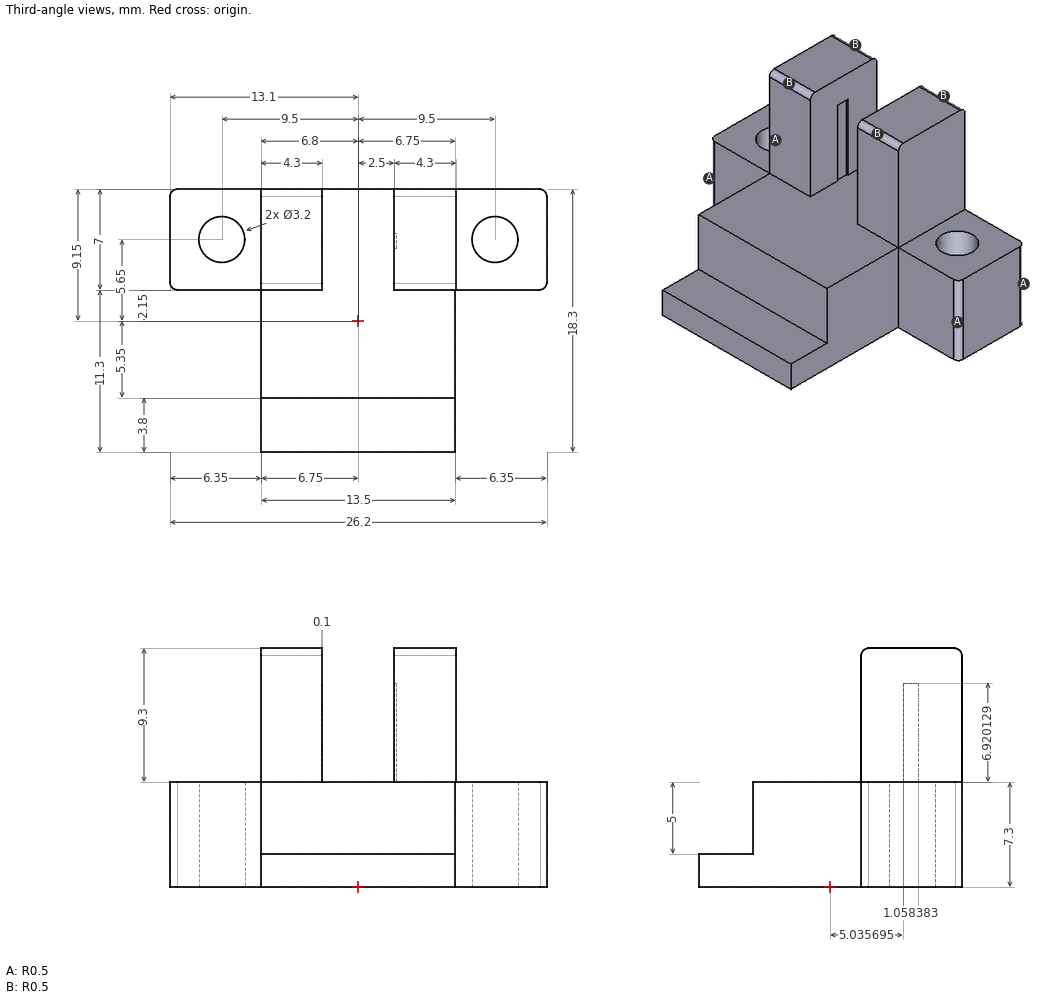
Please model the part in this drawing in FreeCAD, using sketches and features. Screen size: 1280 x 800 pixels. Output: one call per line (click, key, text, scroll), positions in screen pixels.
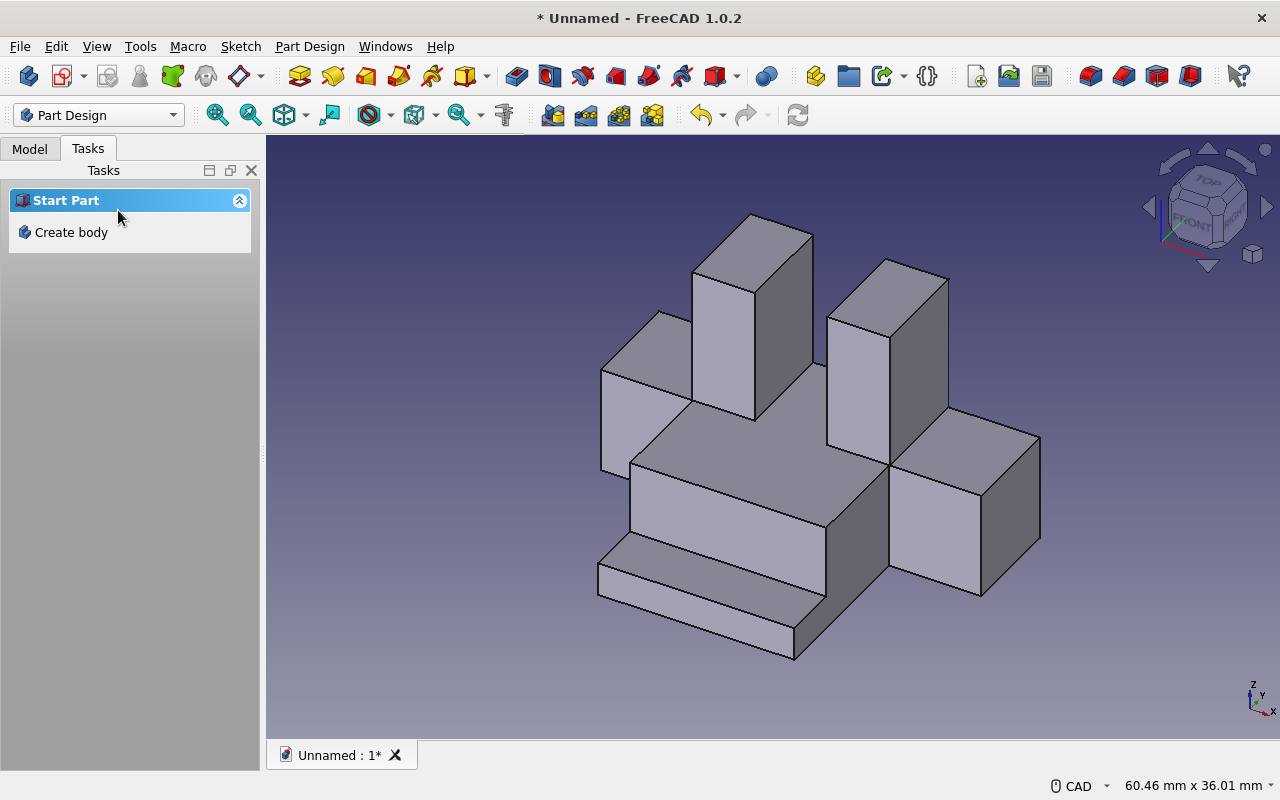
click(772, 451)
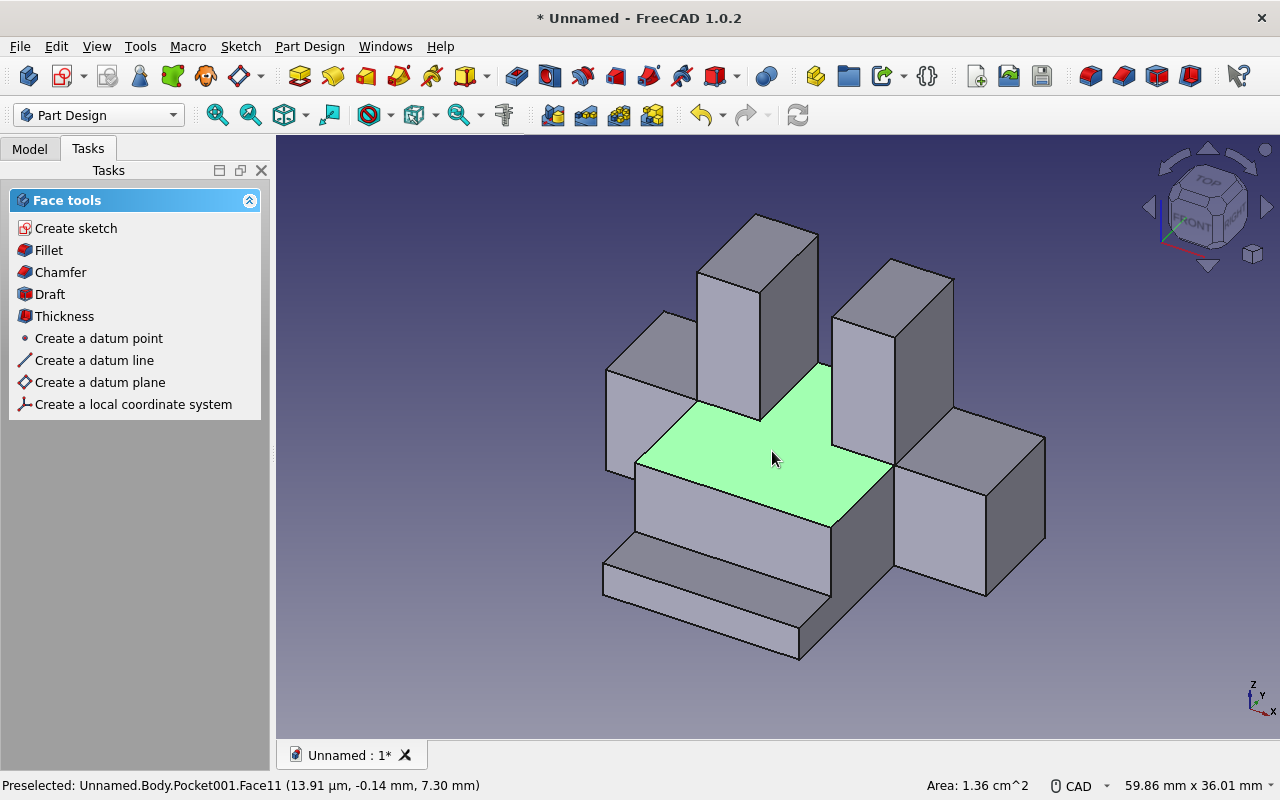
click(62, 76)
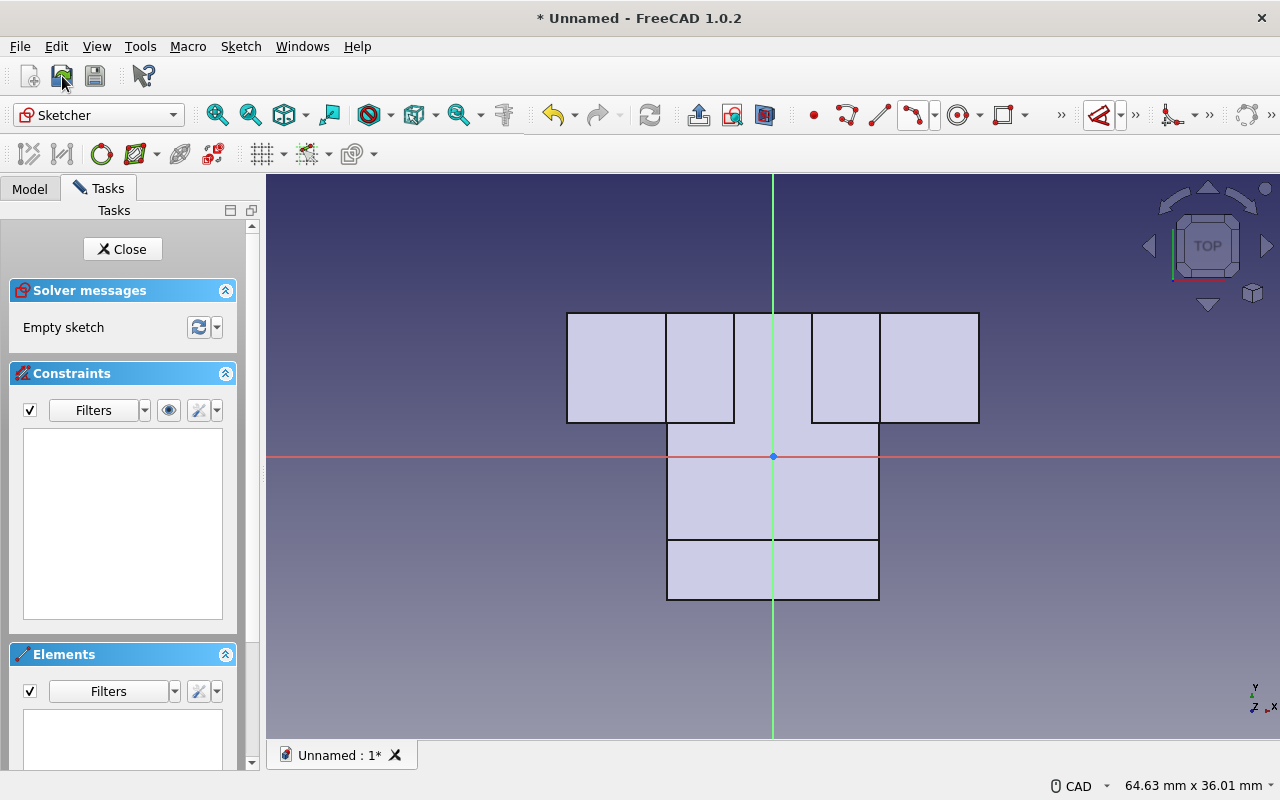
scroll(856, 330, up, 3)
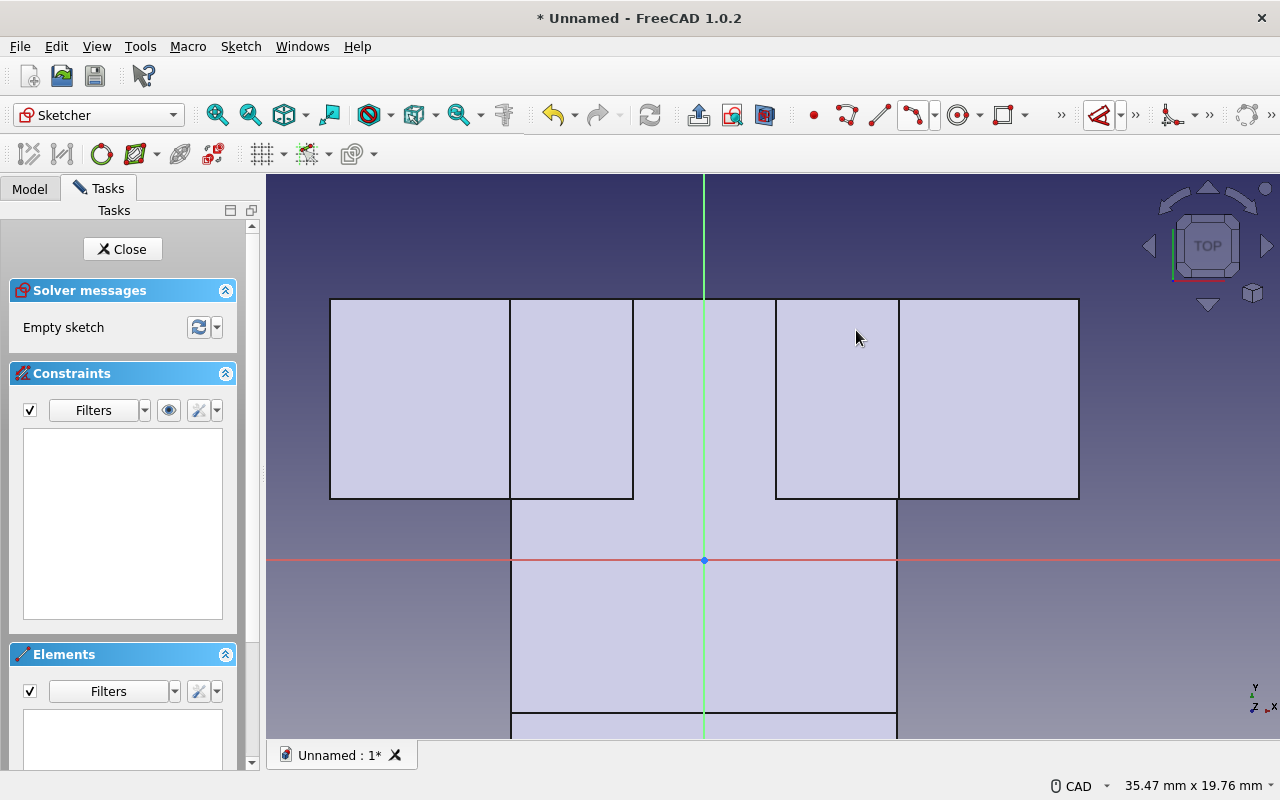
key(g)
key(c)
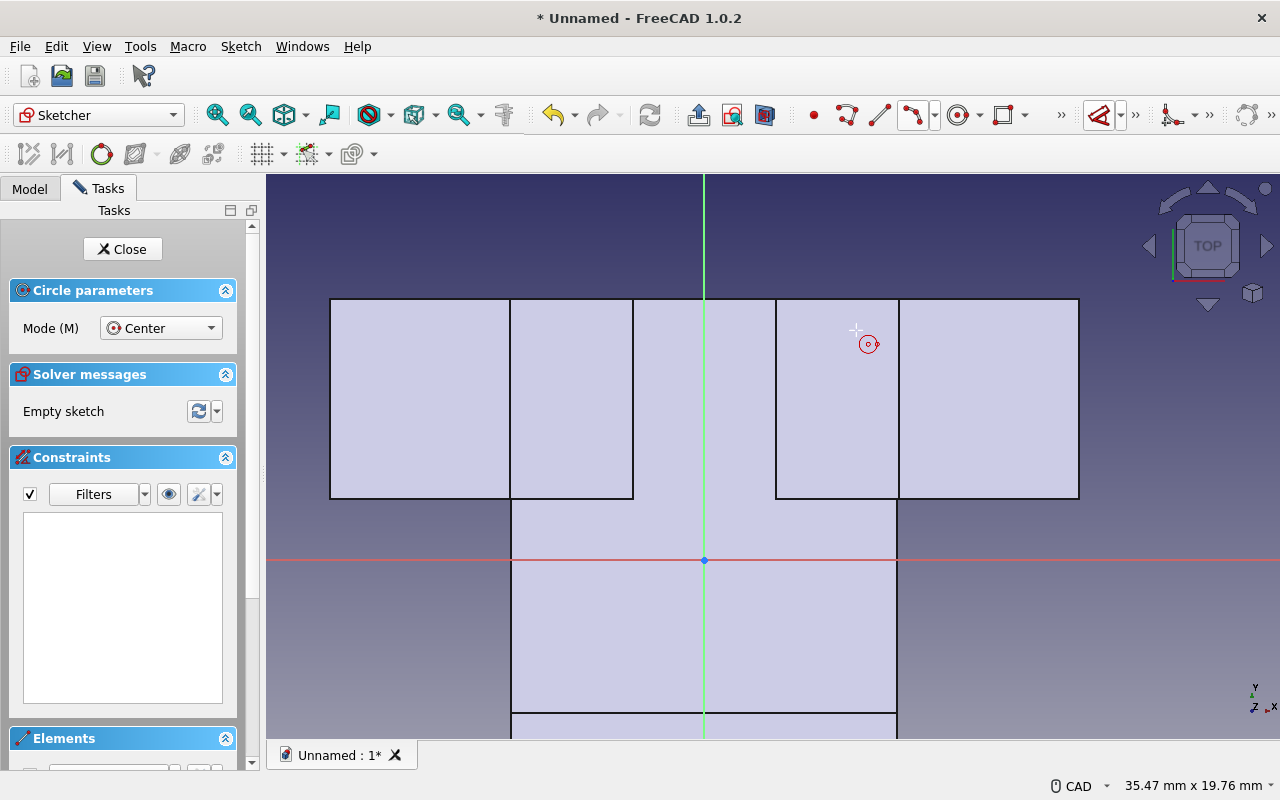
click(433, 399)
click(465, 366)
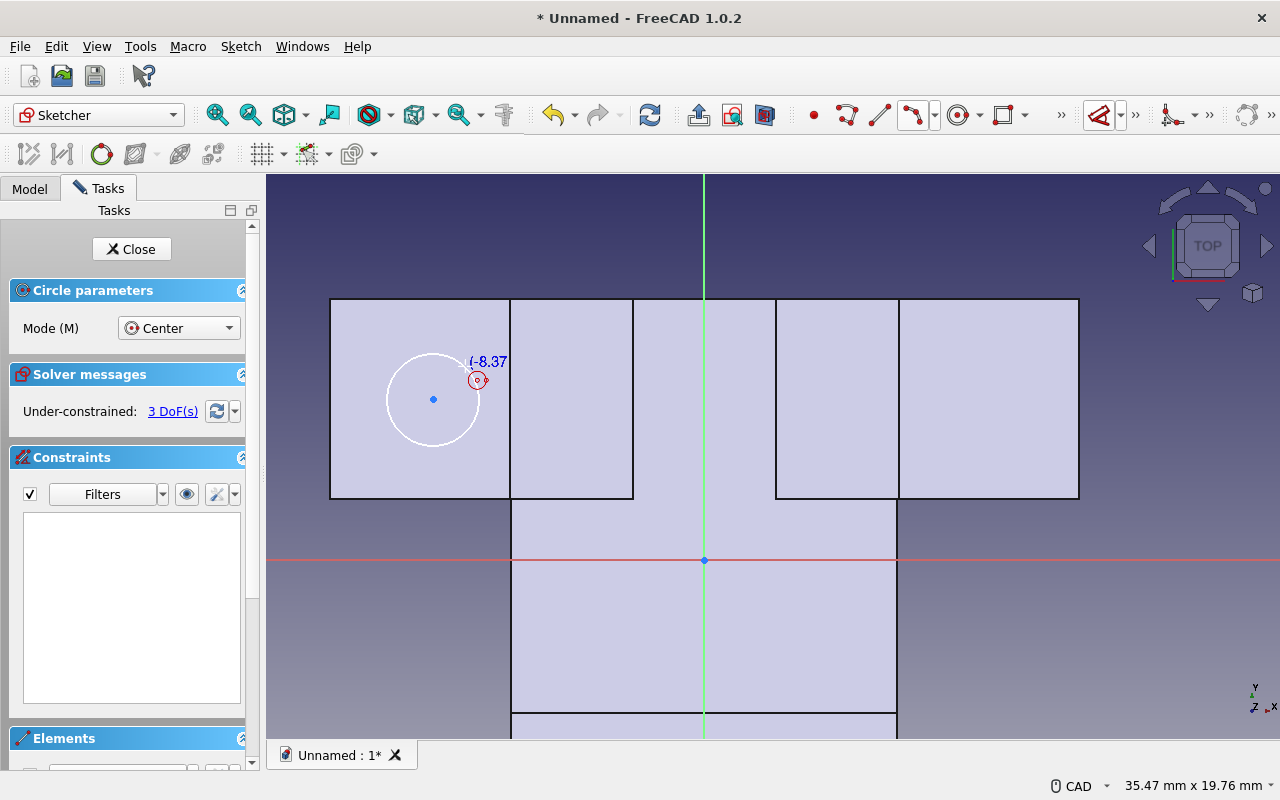
click(976, 399)
click(1008, 366)
key(Escape)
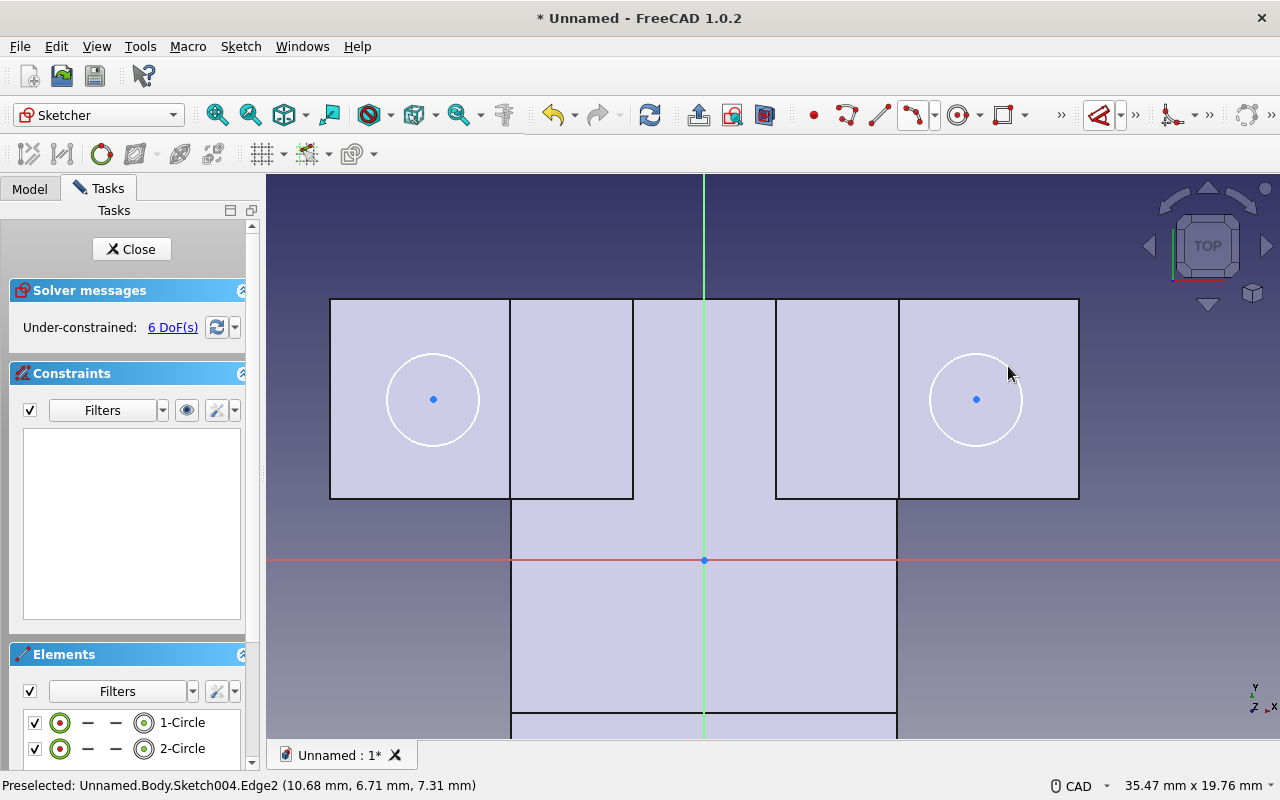
click(465, 367)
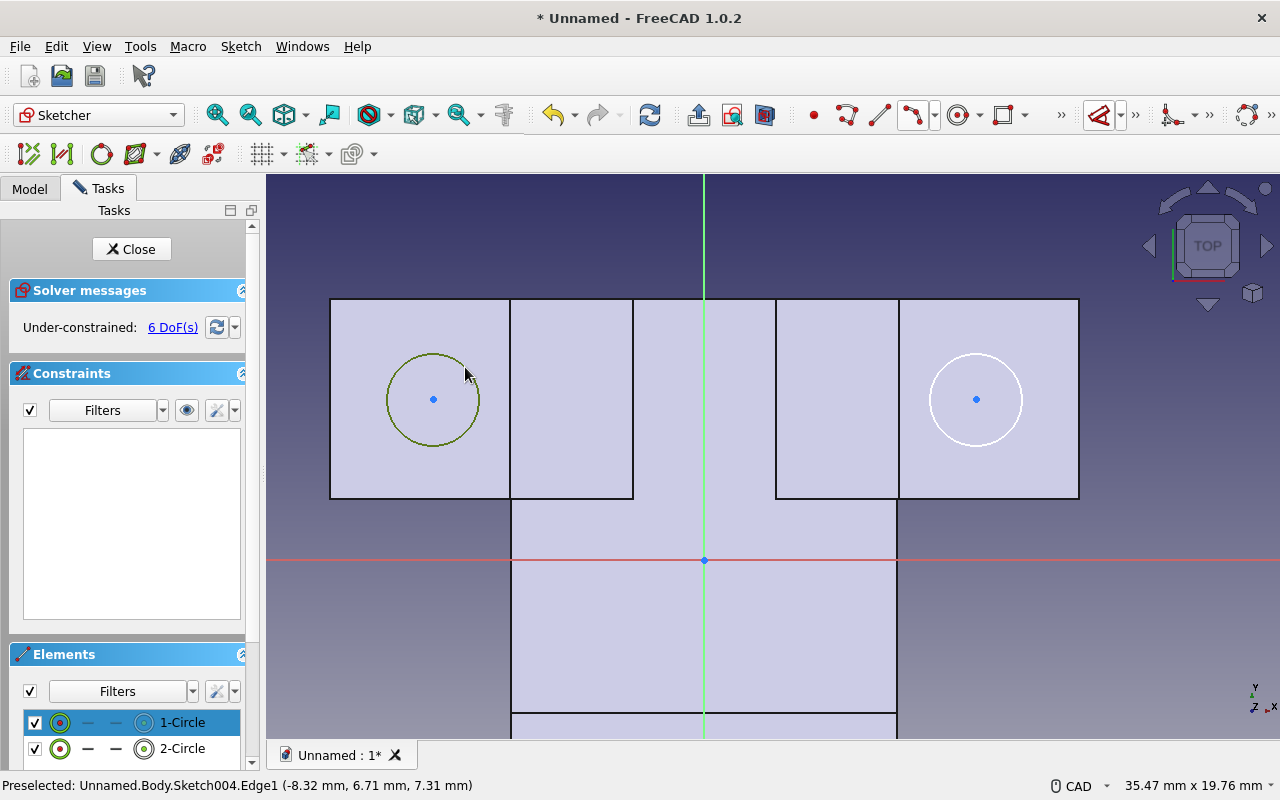
click(1008, 367)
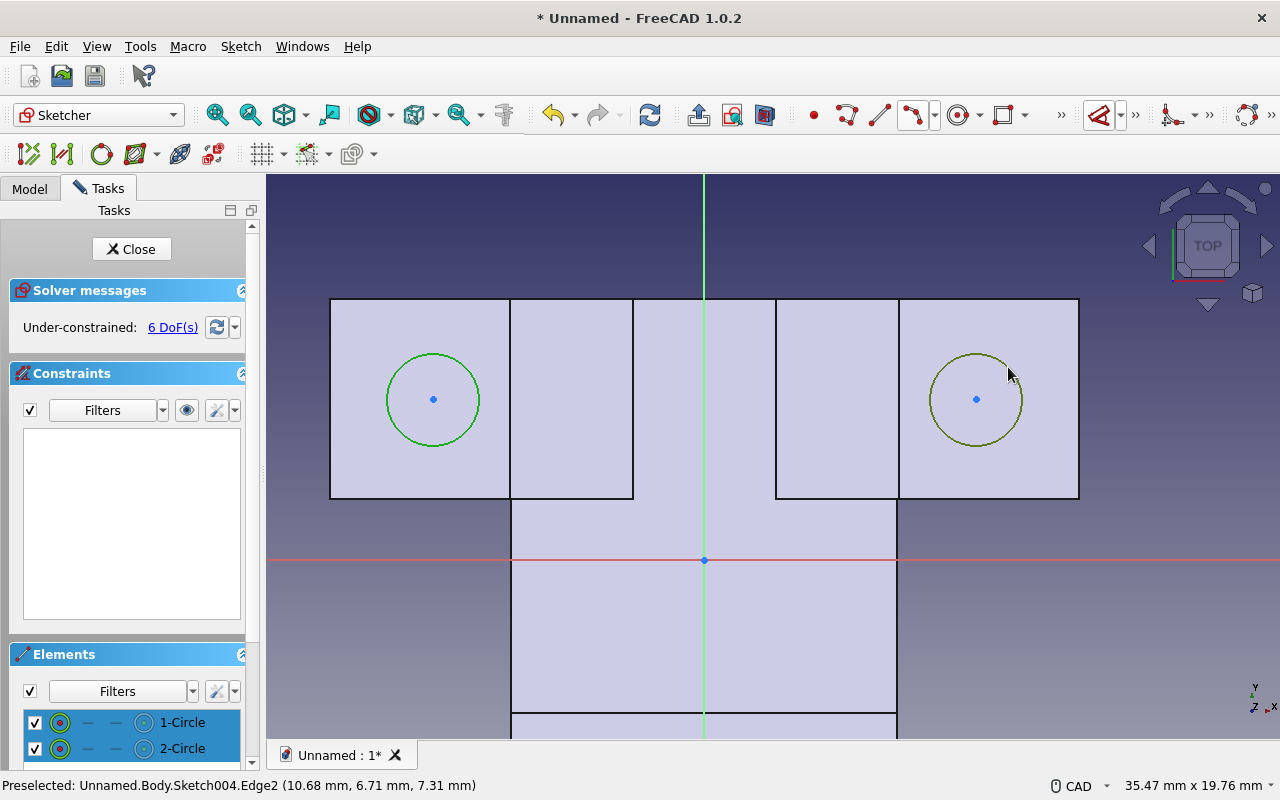
key(e)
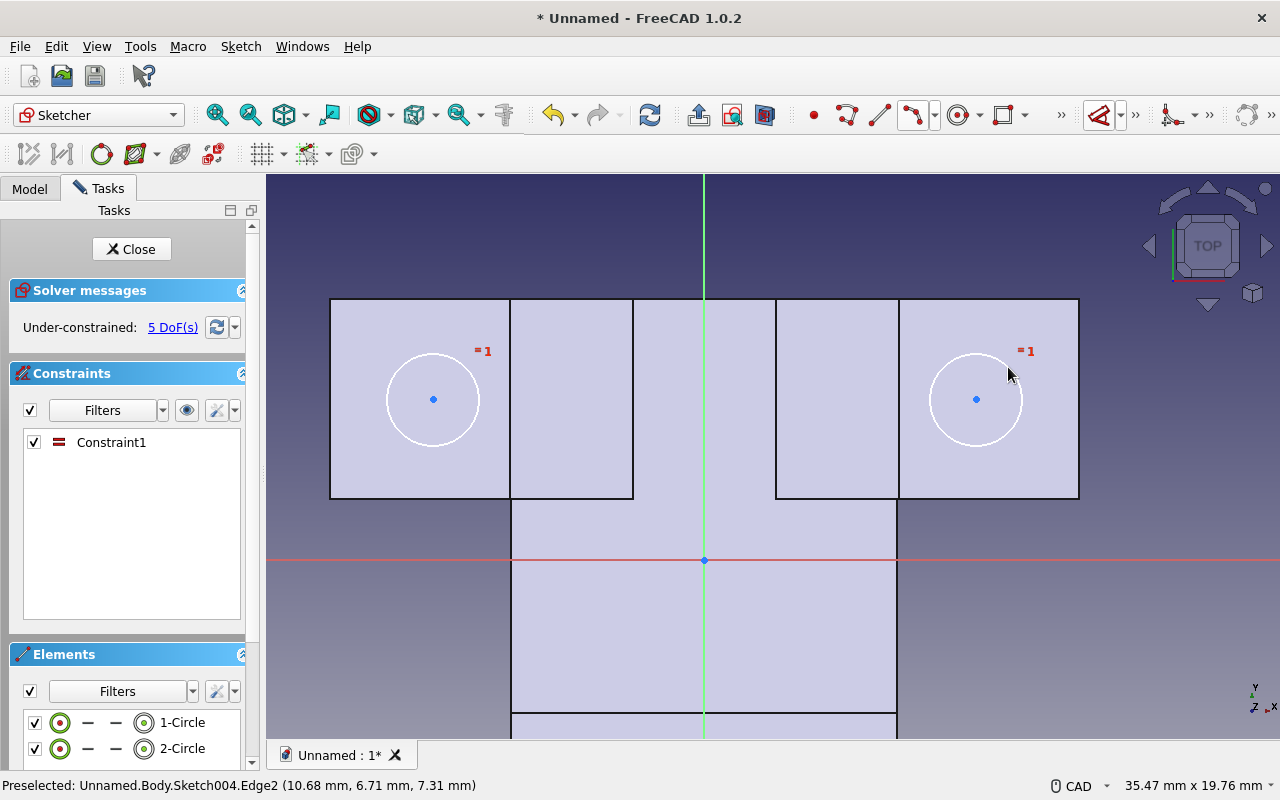
click(433, 400)